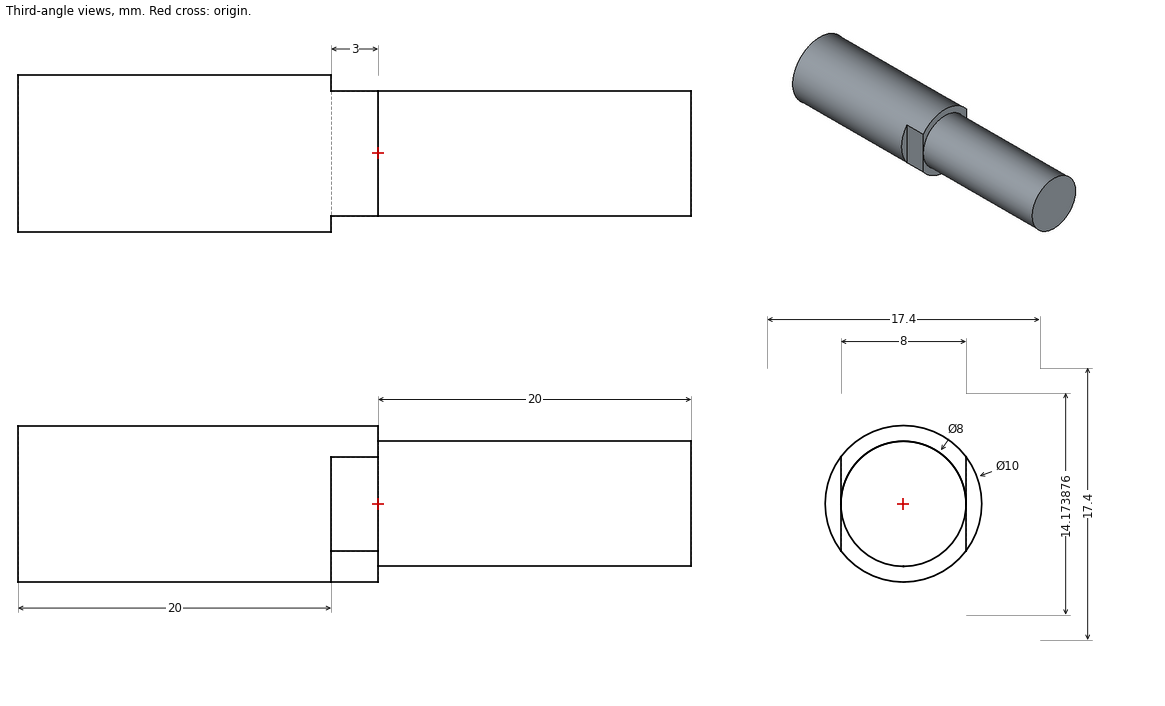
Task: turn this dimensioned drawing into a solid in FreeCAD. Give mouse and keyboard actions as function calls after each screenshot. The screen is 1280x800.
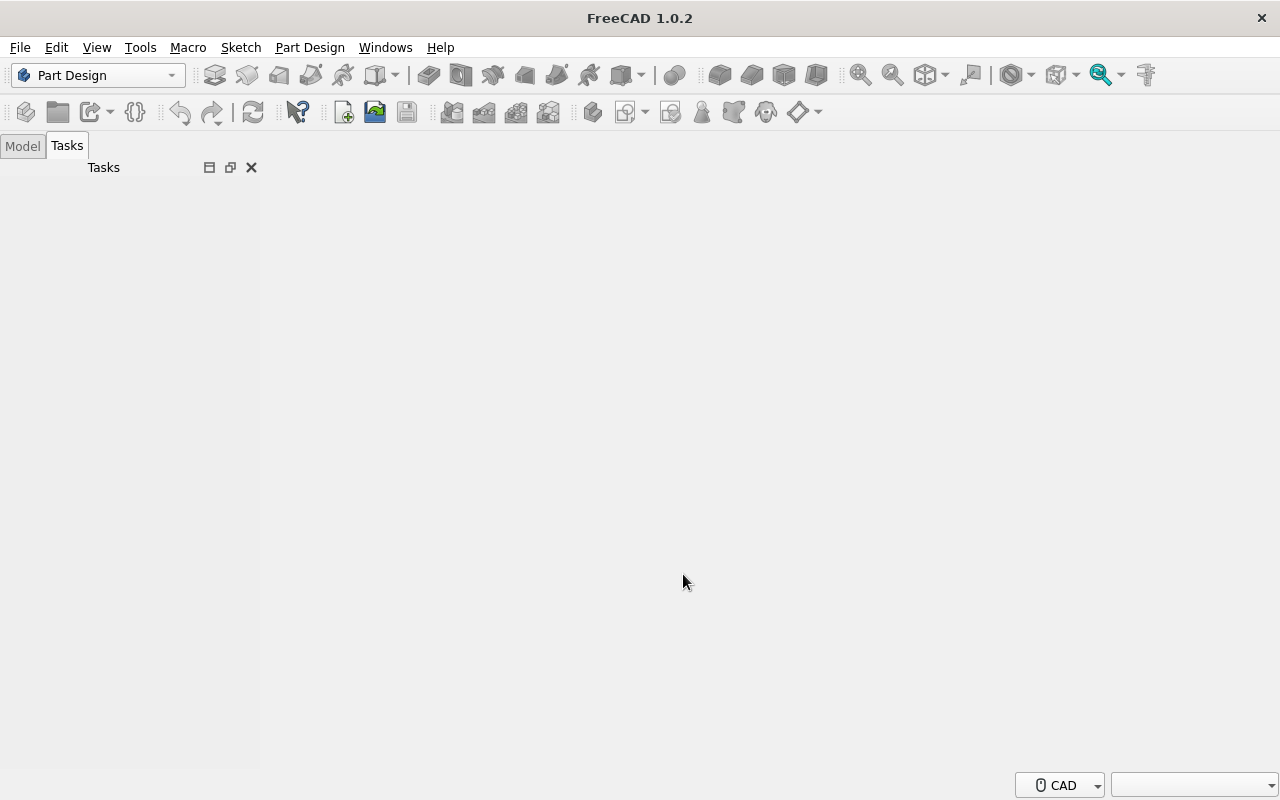
key(ctrl+n)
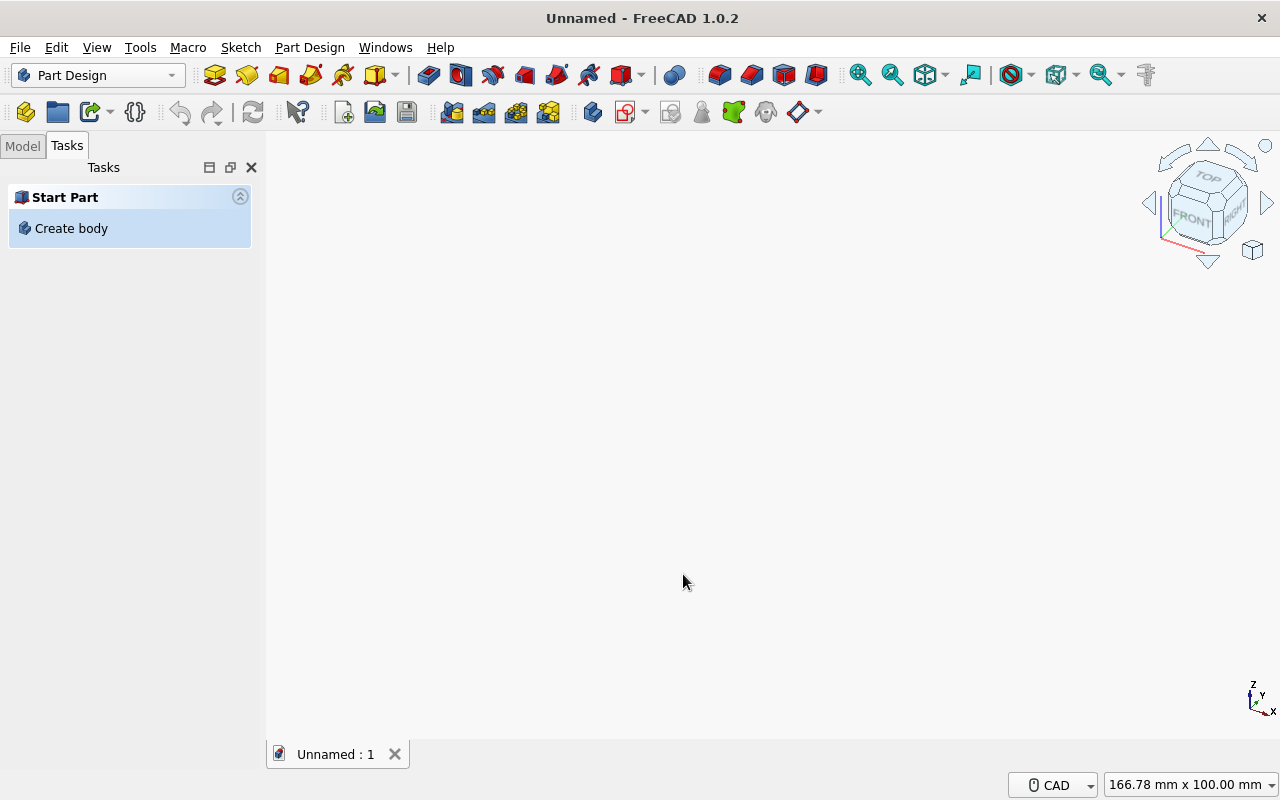
click(626, 112)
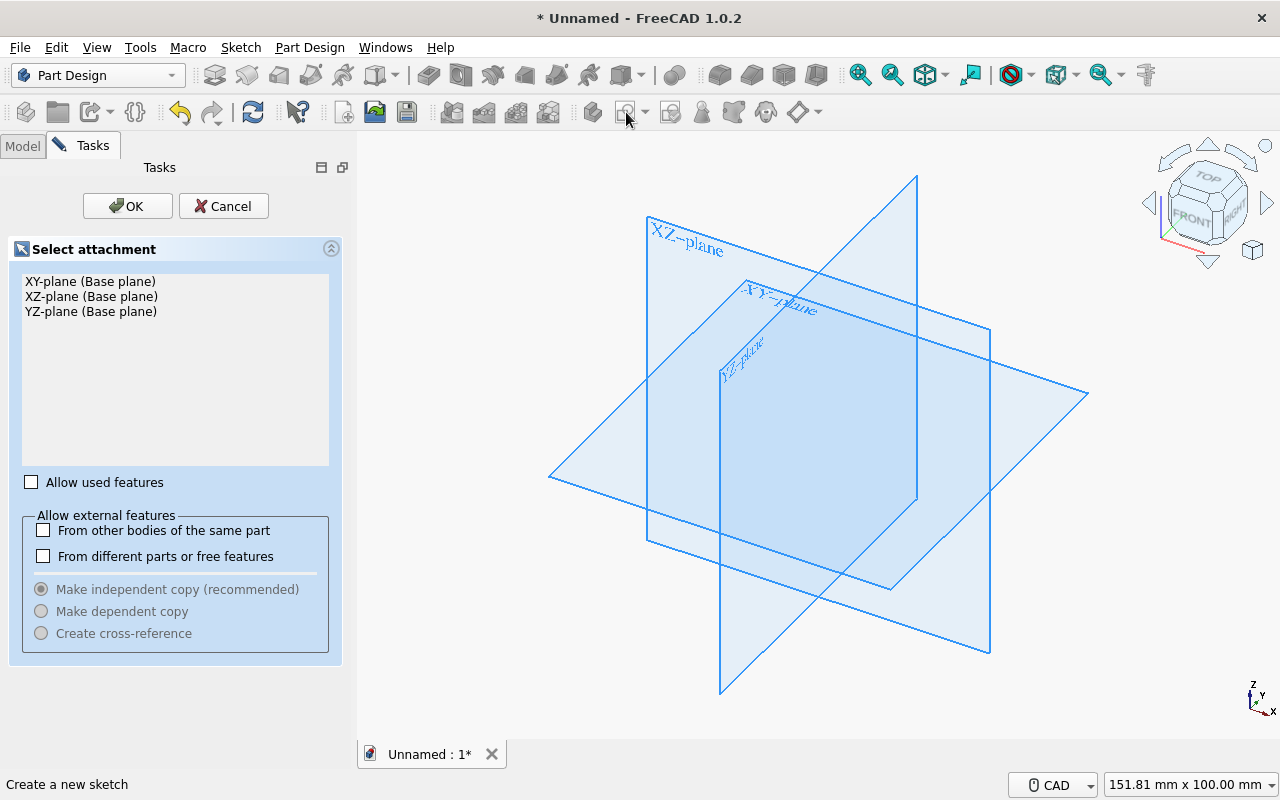
click(82, 312)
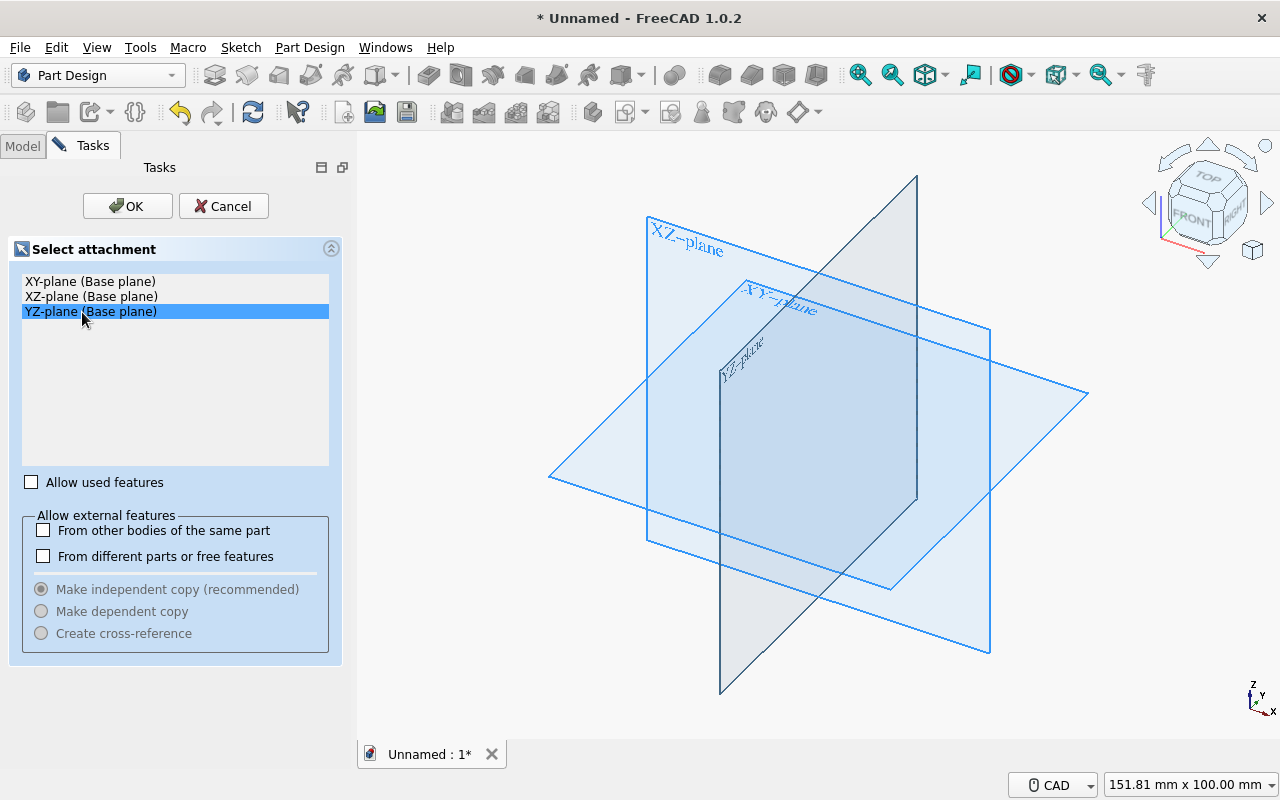
click(128, 206)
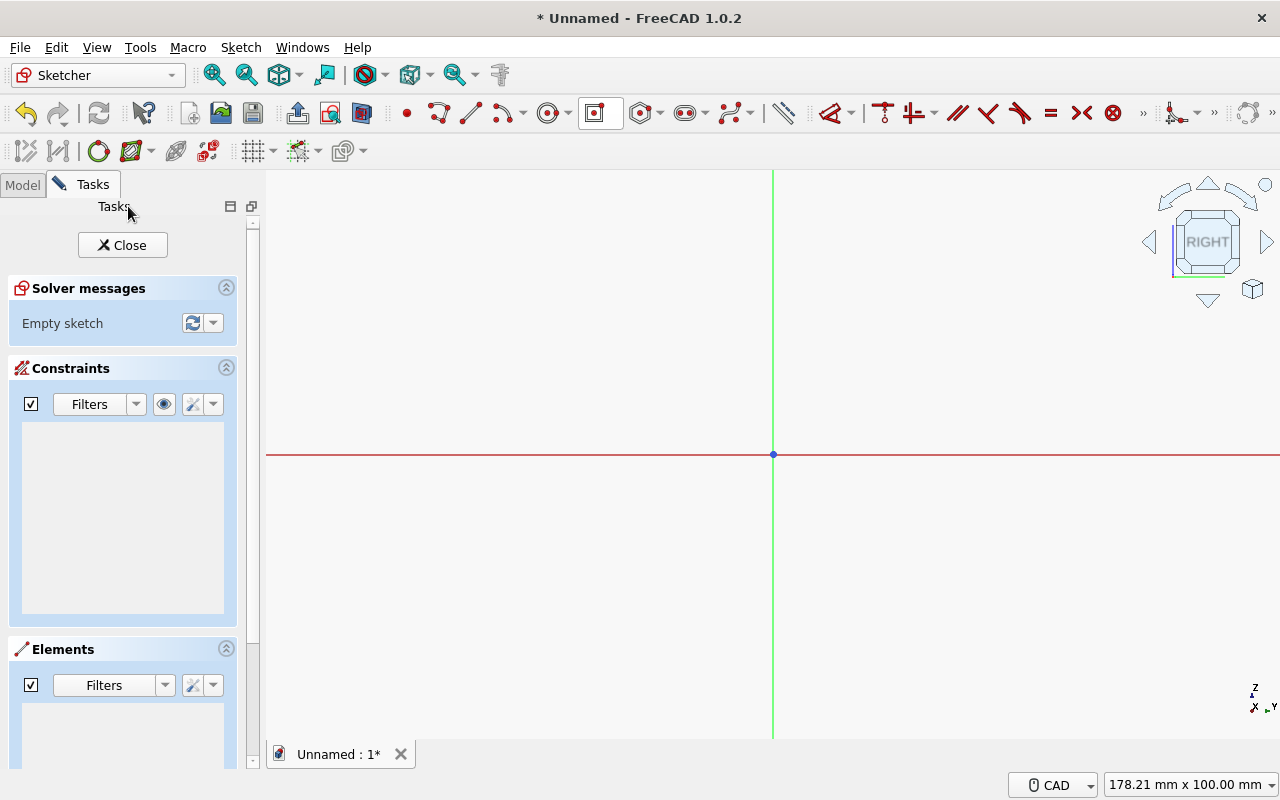
scroll(784, 454, up, 10)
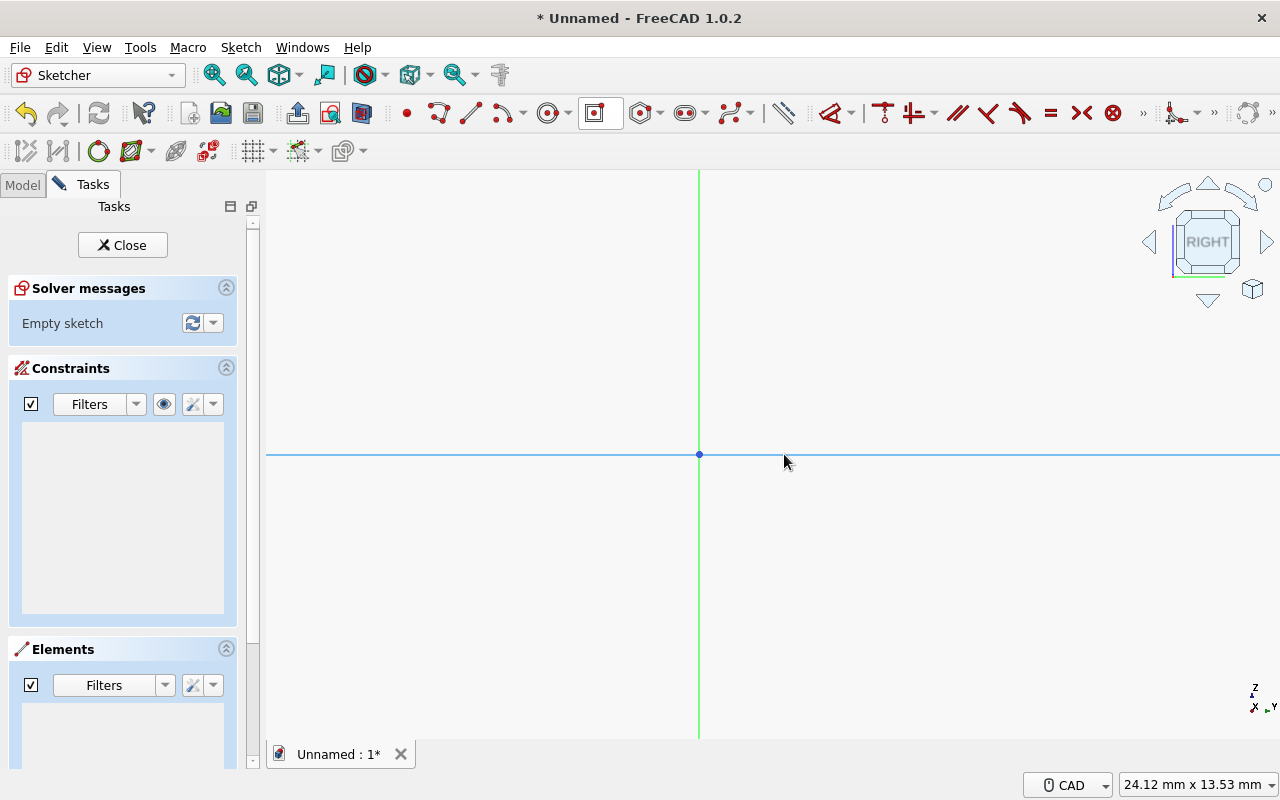
key(g)
key(c)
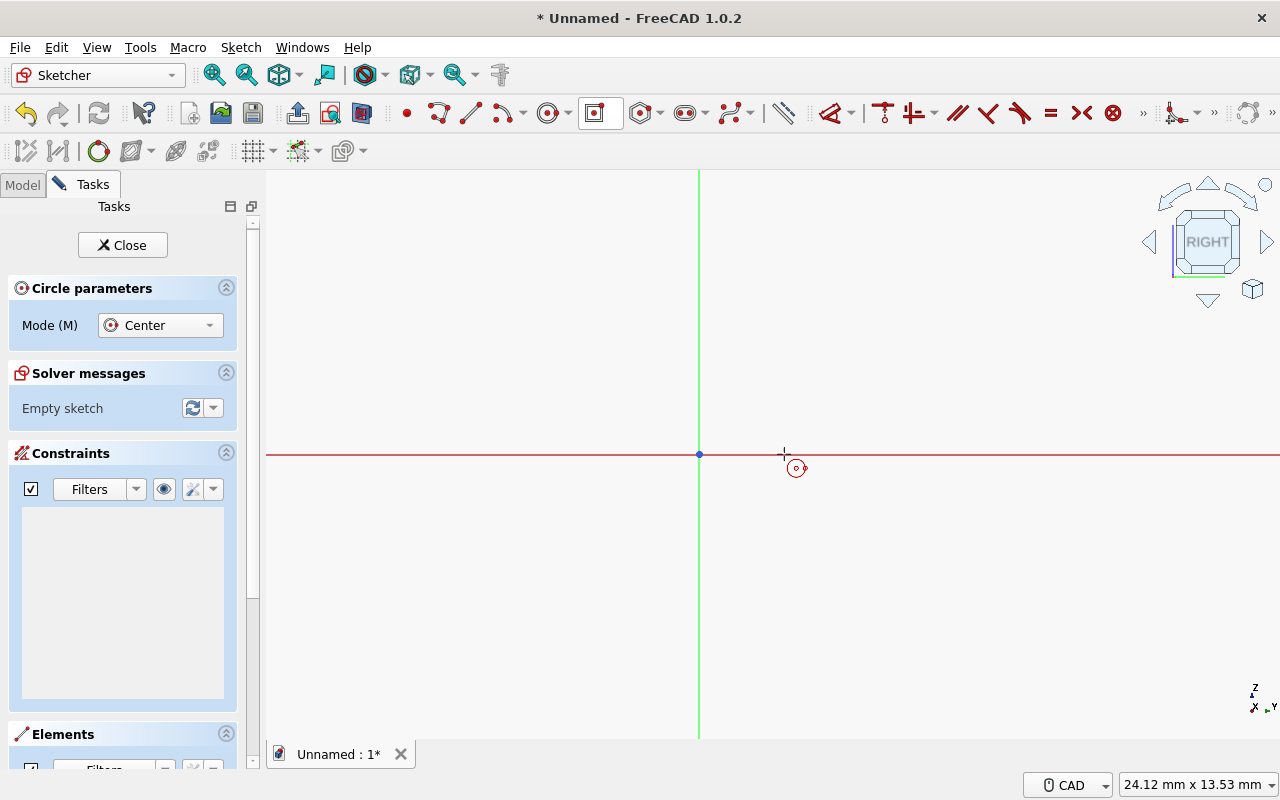
click(699, 454)
click(818, 336)
key(Escape)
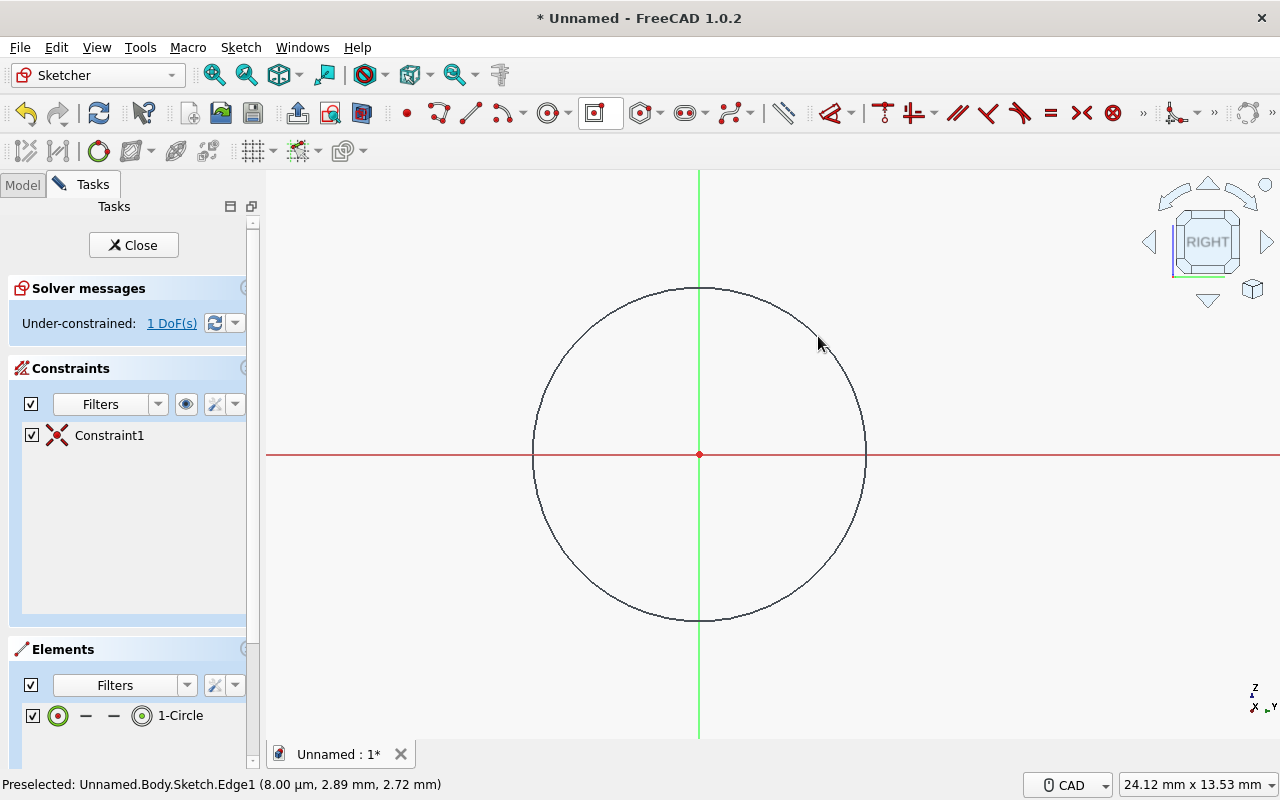
click(817, 336)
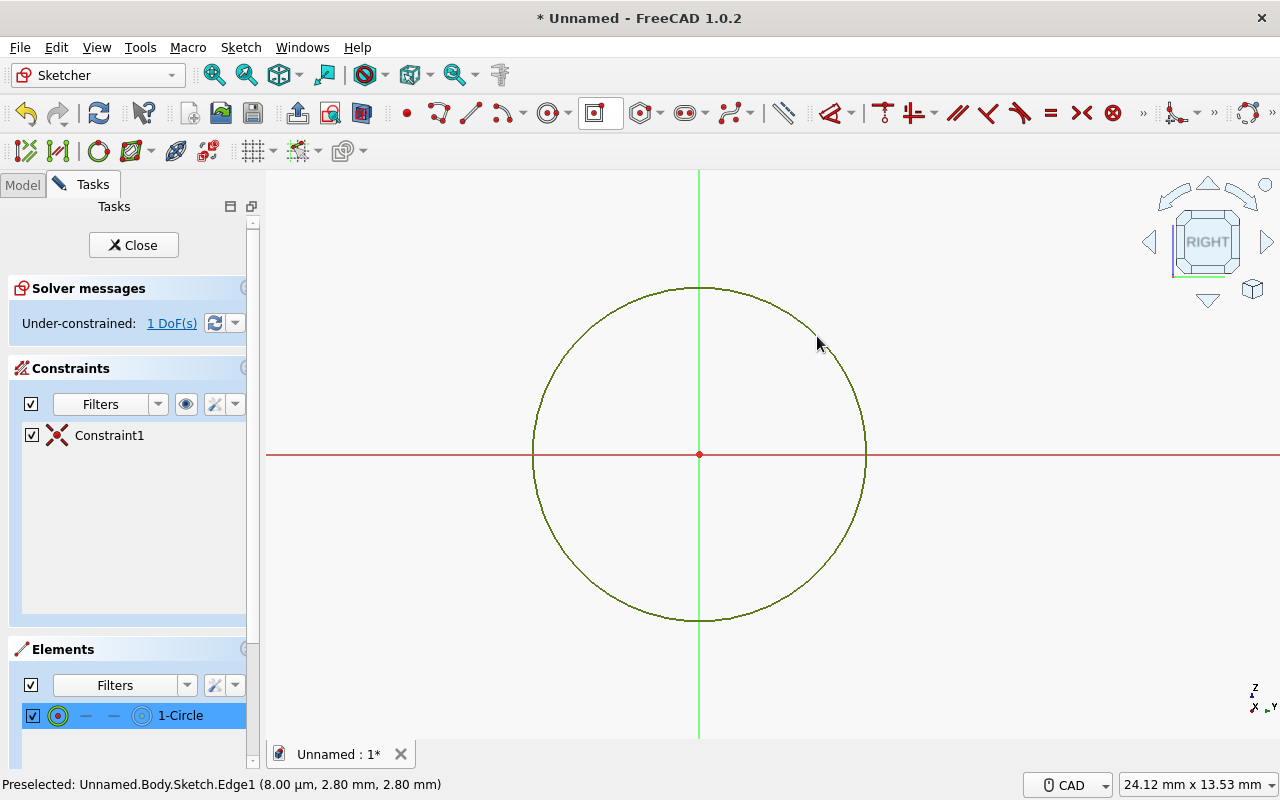
key(k)
key(o)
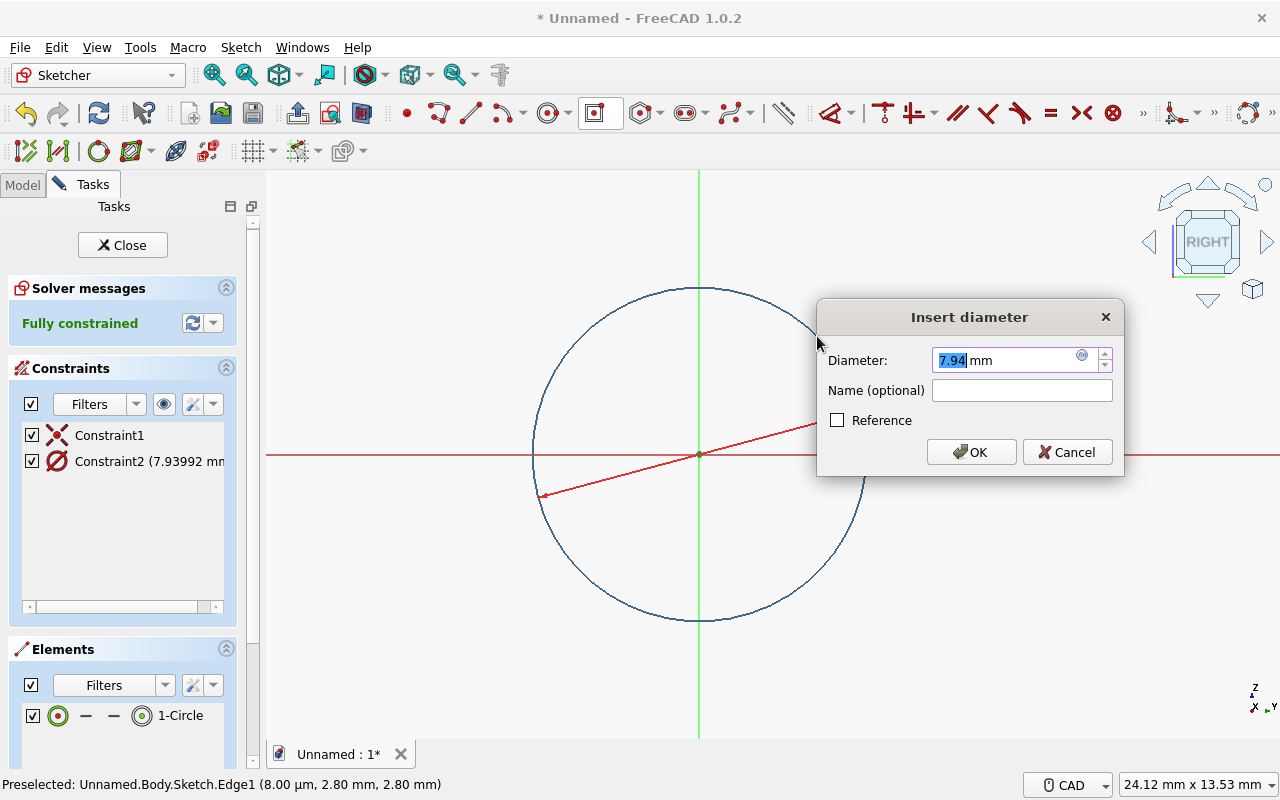
text(8)
key(Return)